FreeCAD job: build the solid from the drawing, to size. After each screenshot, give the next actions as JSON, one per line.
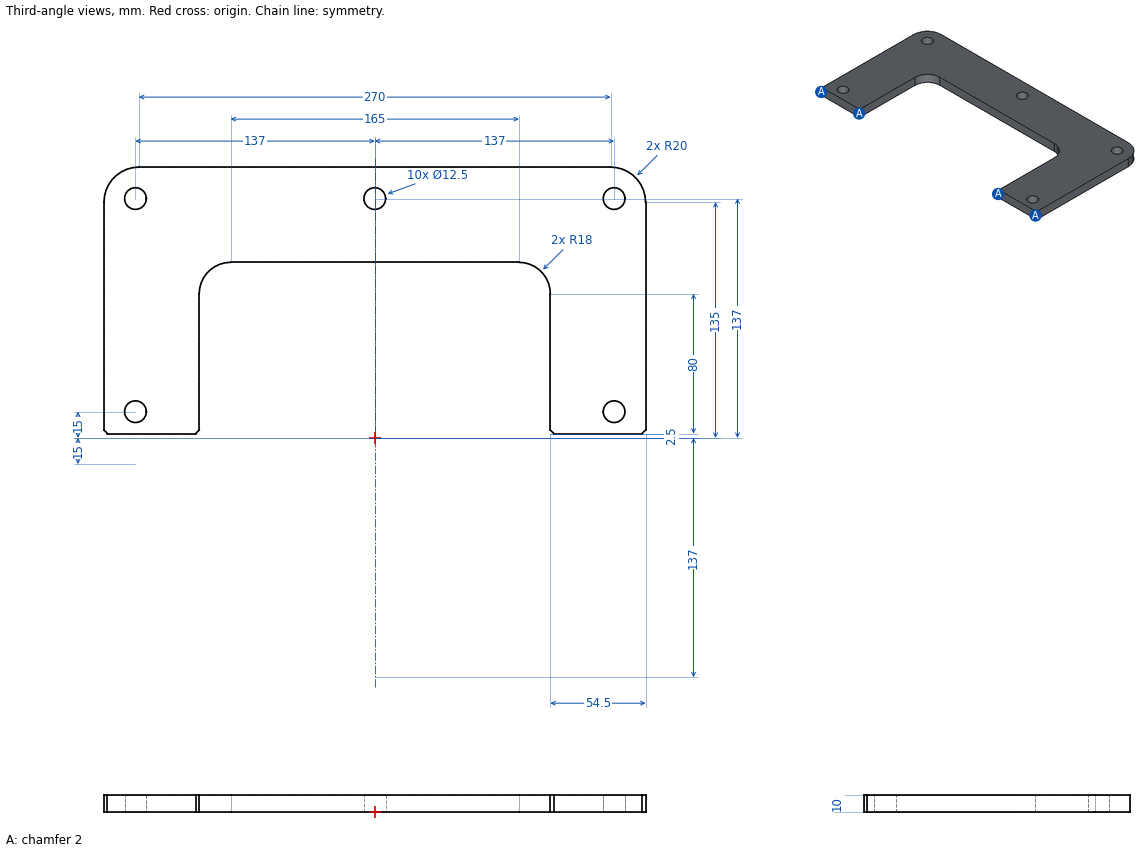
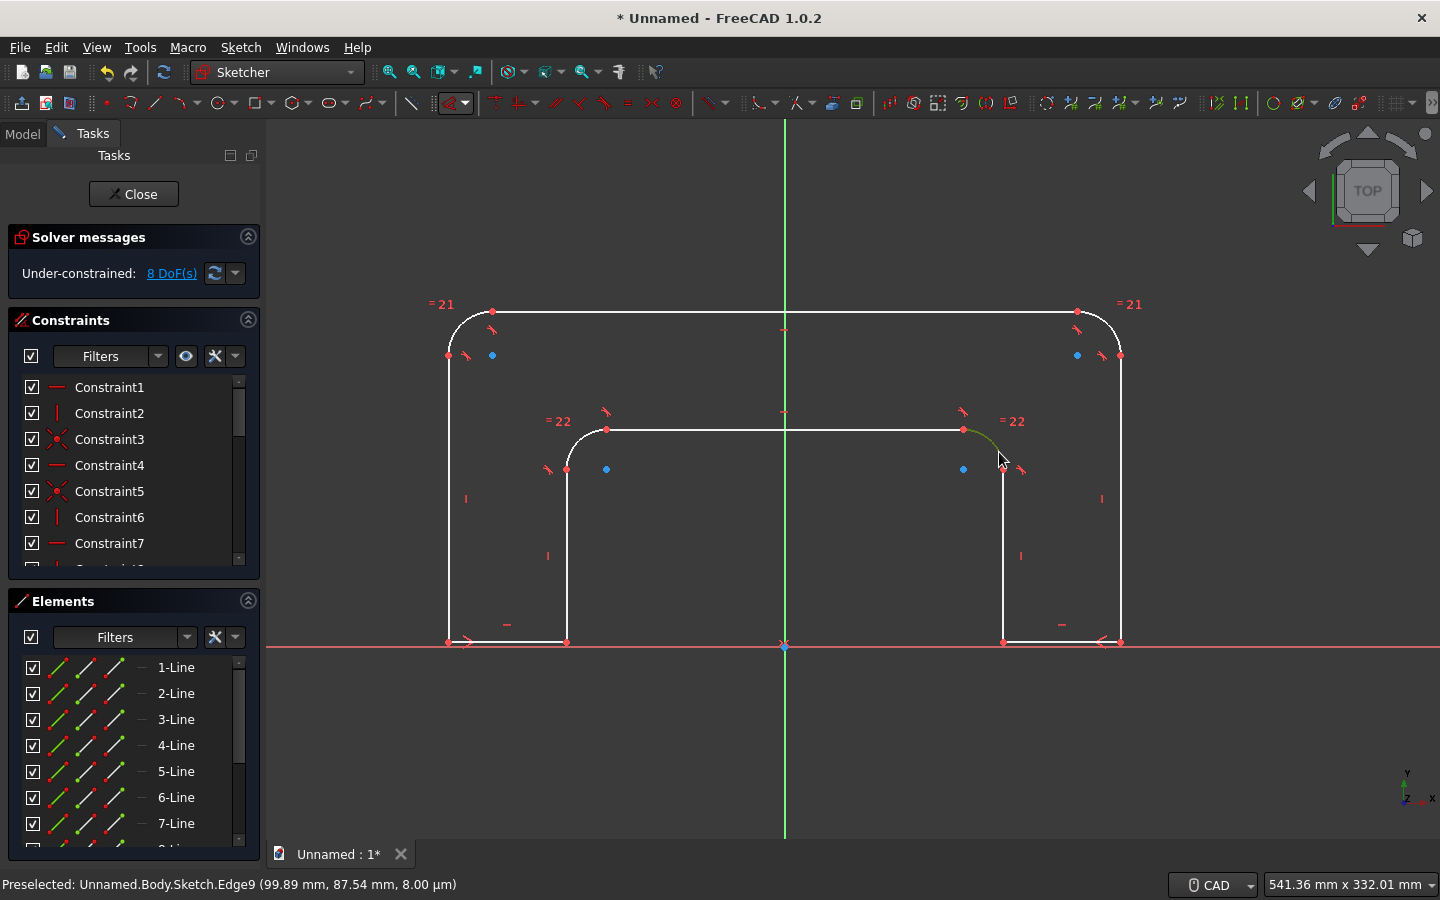
{"action": "left_click", "coordinate": [468, 104]}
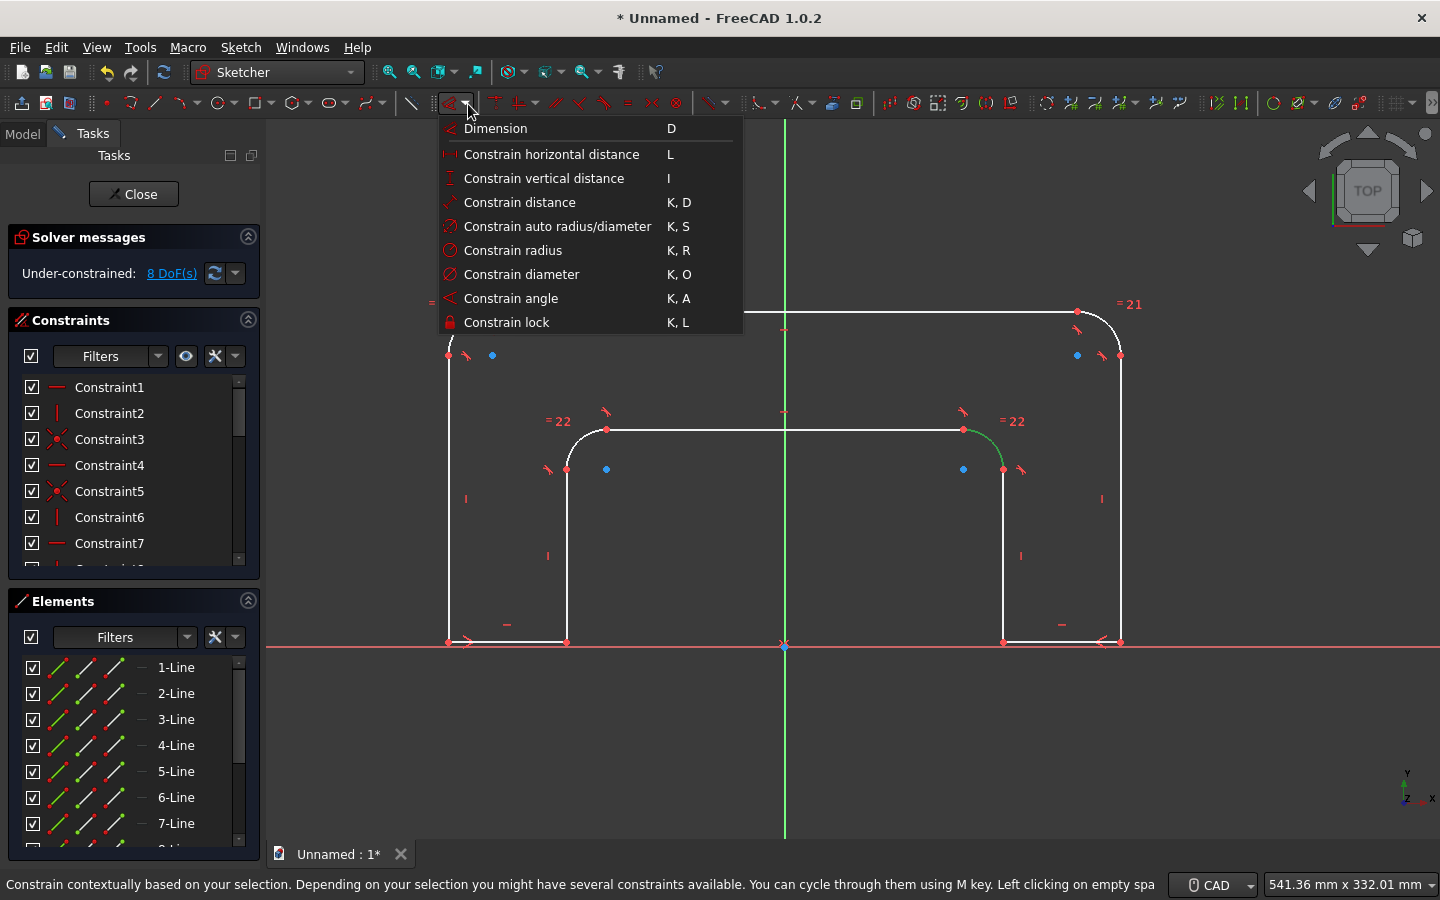
{"action": "left_click", "coordinate": [591, 250]}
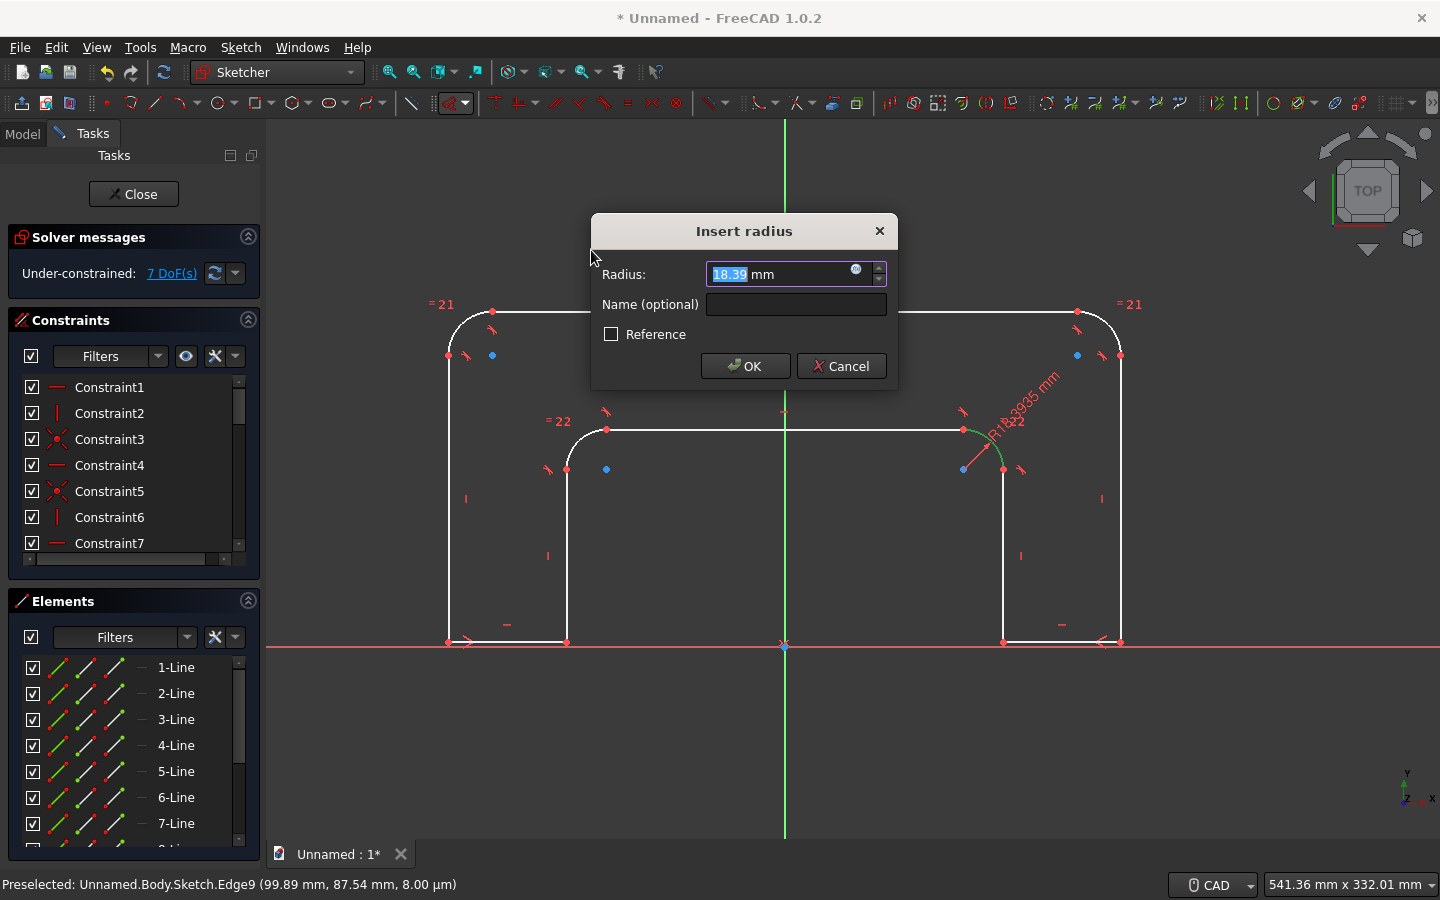
{"action": "type", "text": "18"}
{"action": "key", "text": "Return"}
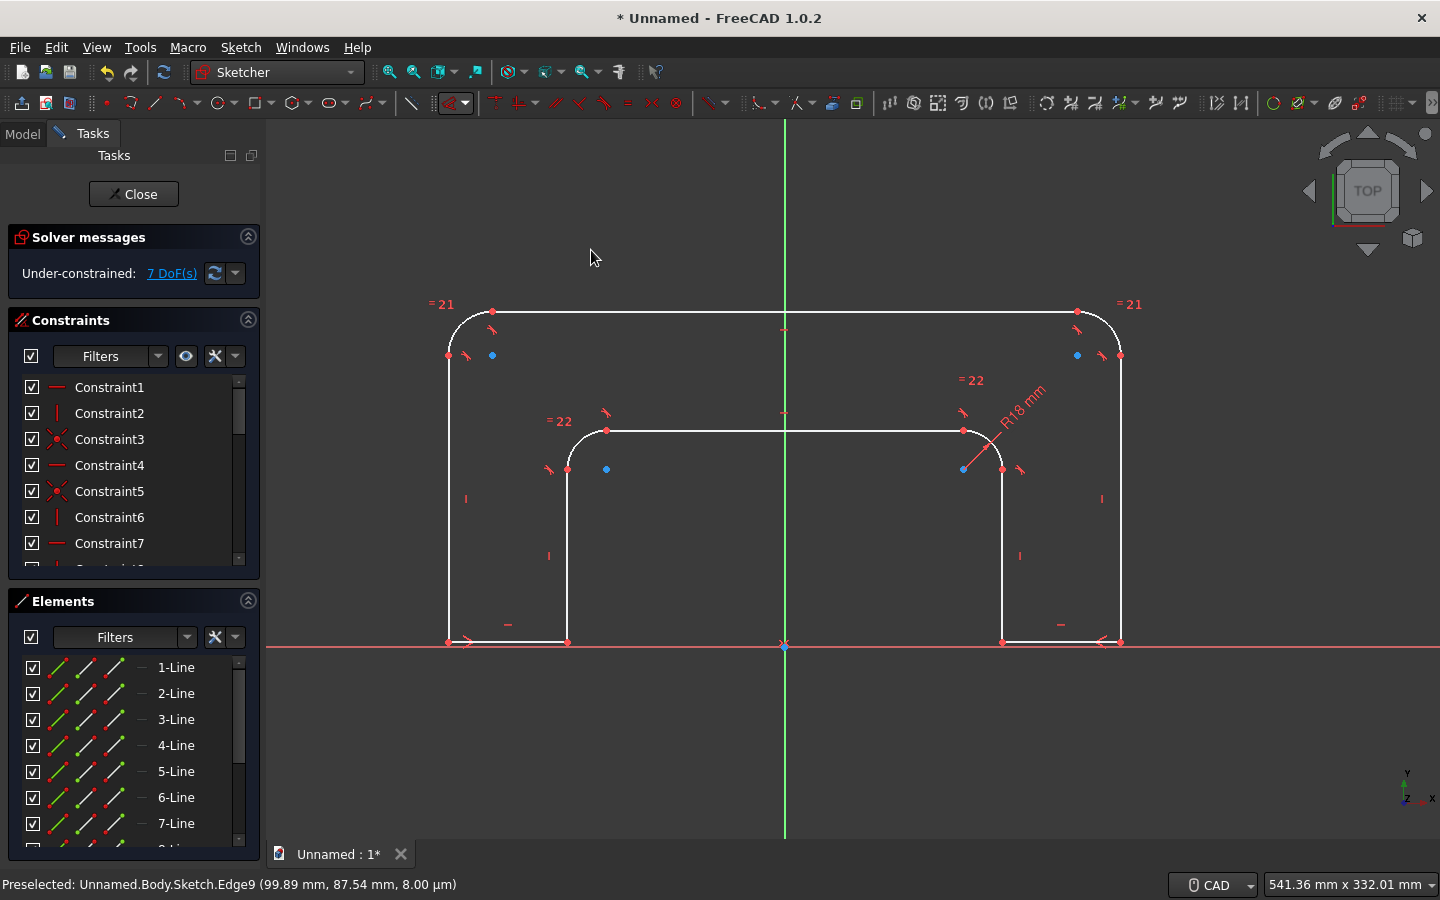
{"action": "left_click", "coordinate": [1116, 336]}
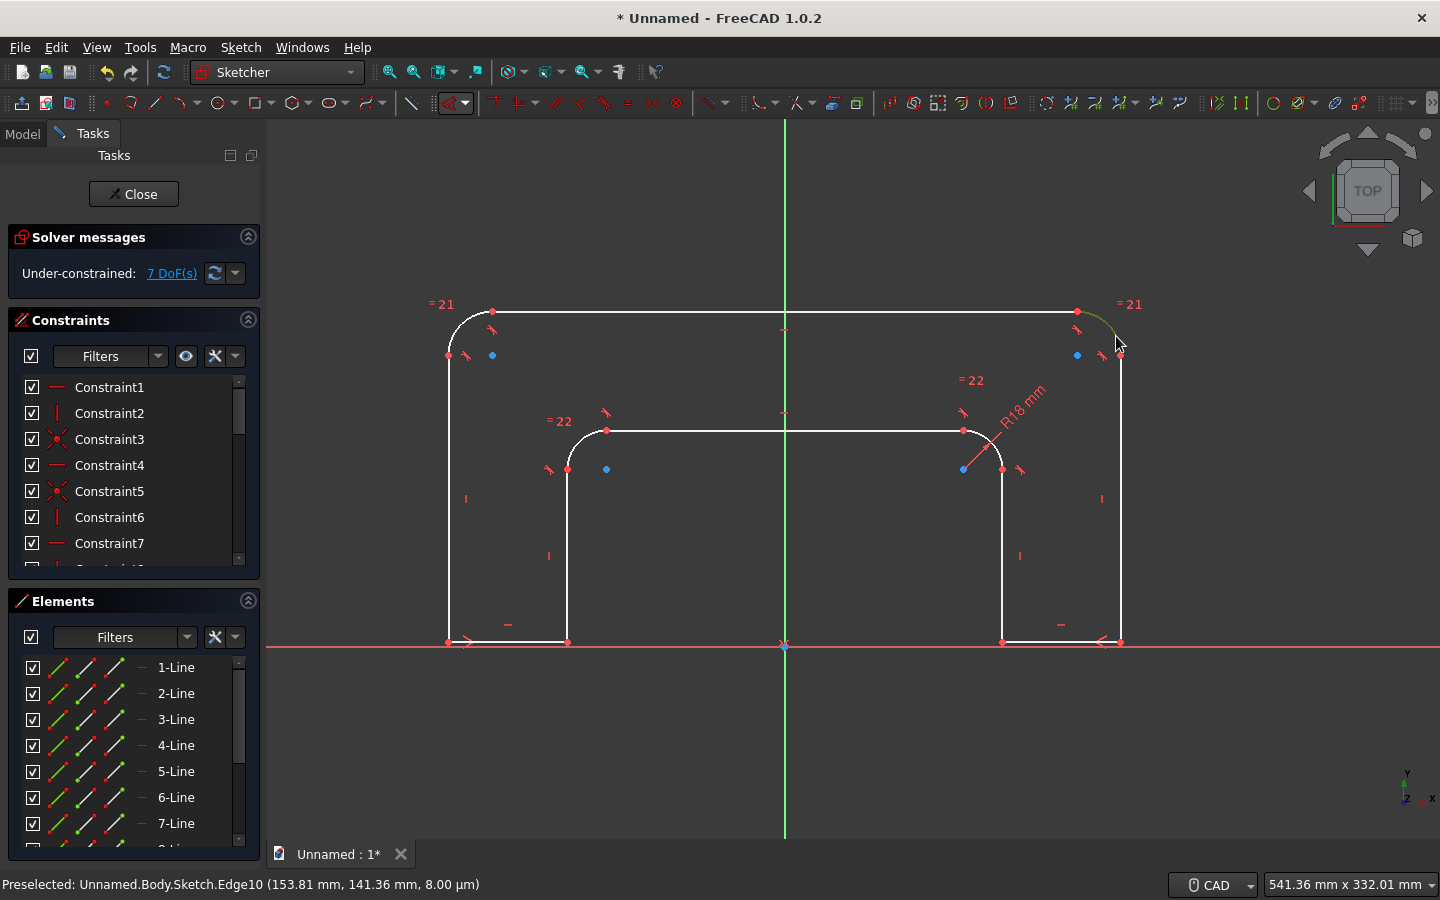
{"action": "key", "text": "k r"}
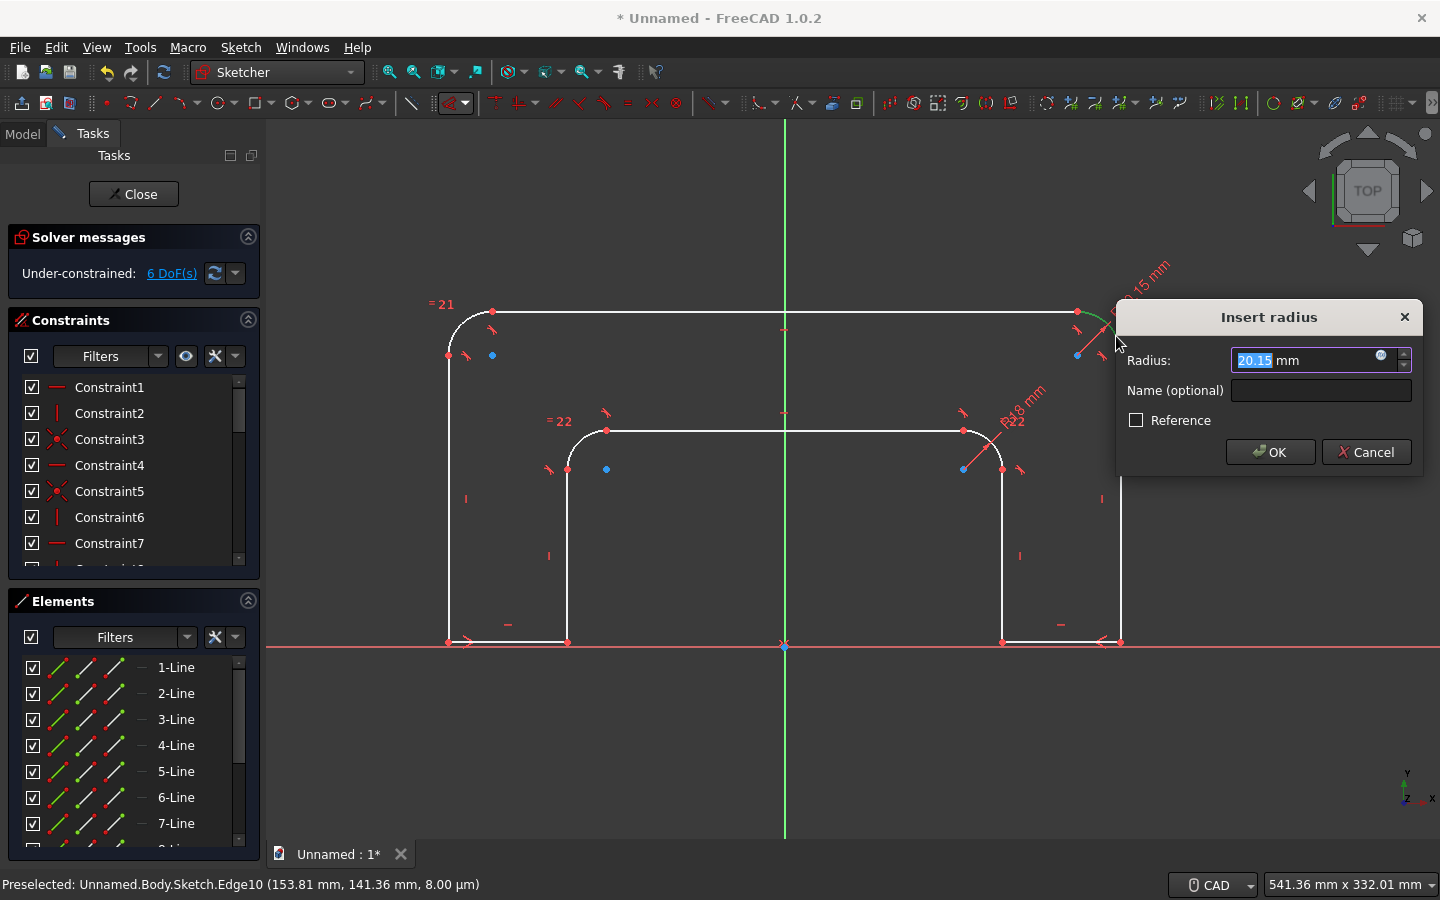
{"action": "type", "text": "20"}
{"action": "key", "text": "Return"}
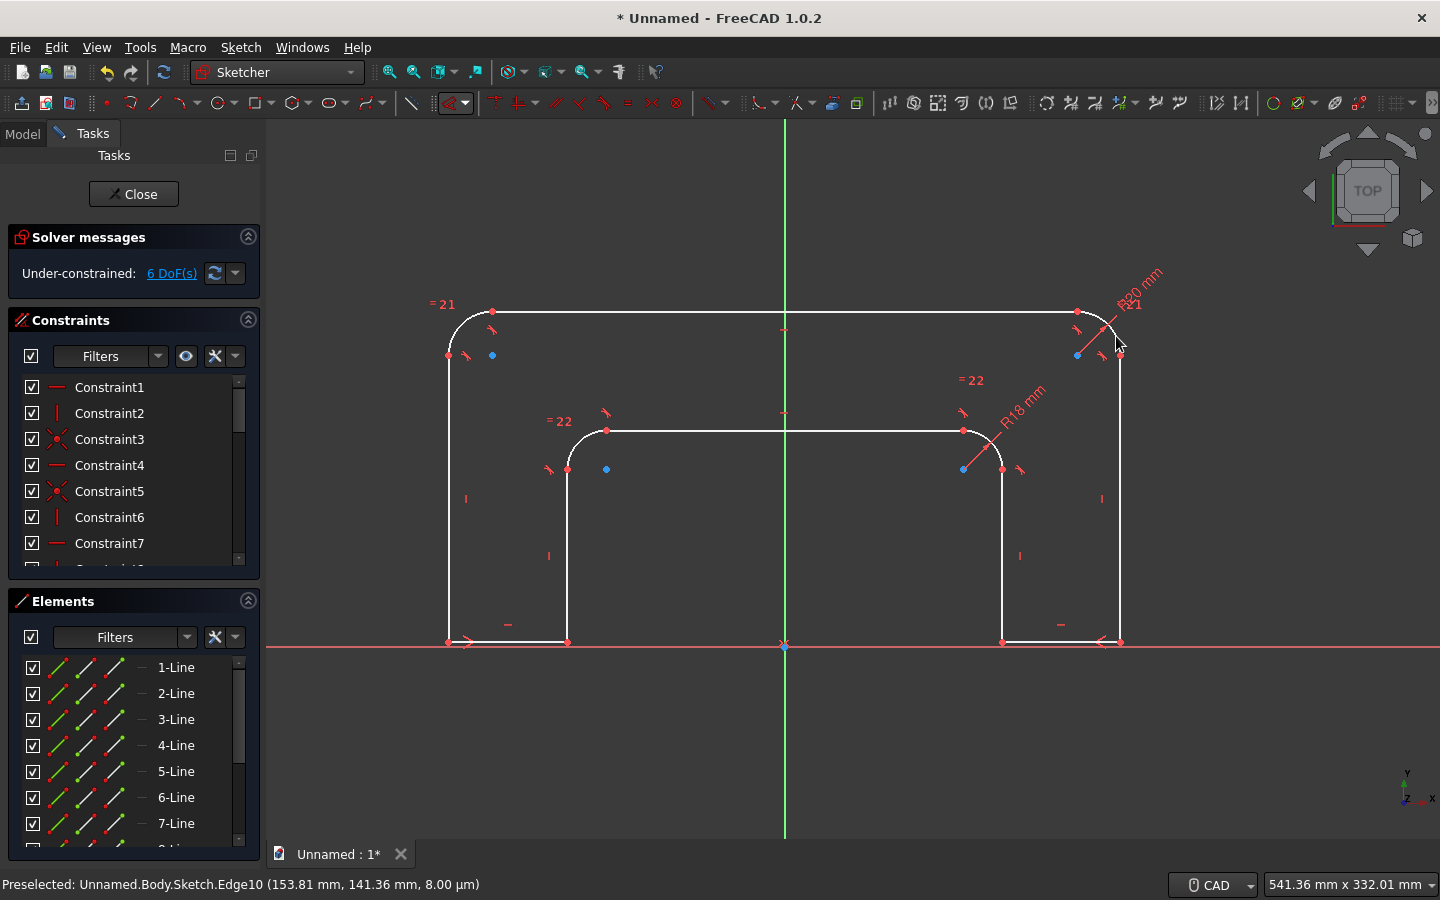
{"action": "left_click", "coordinate": [1002, 521]}